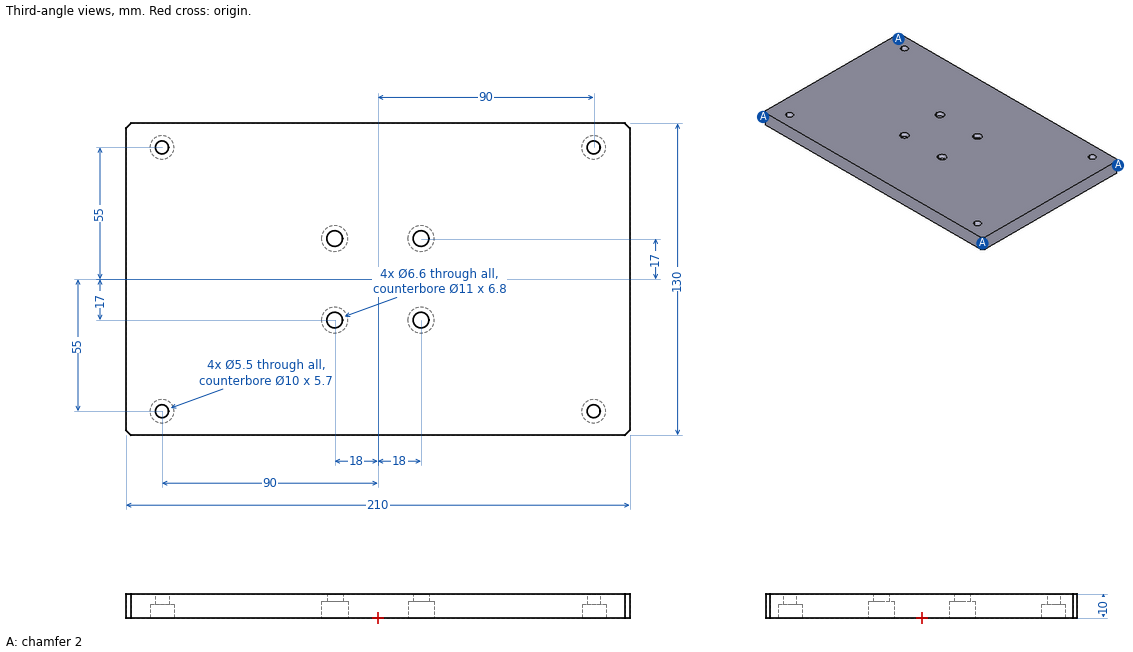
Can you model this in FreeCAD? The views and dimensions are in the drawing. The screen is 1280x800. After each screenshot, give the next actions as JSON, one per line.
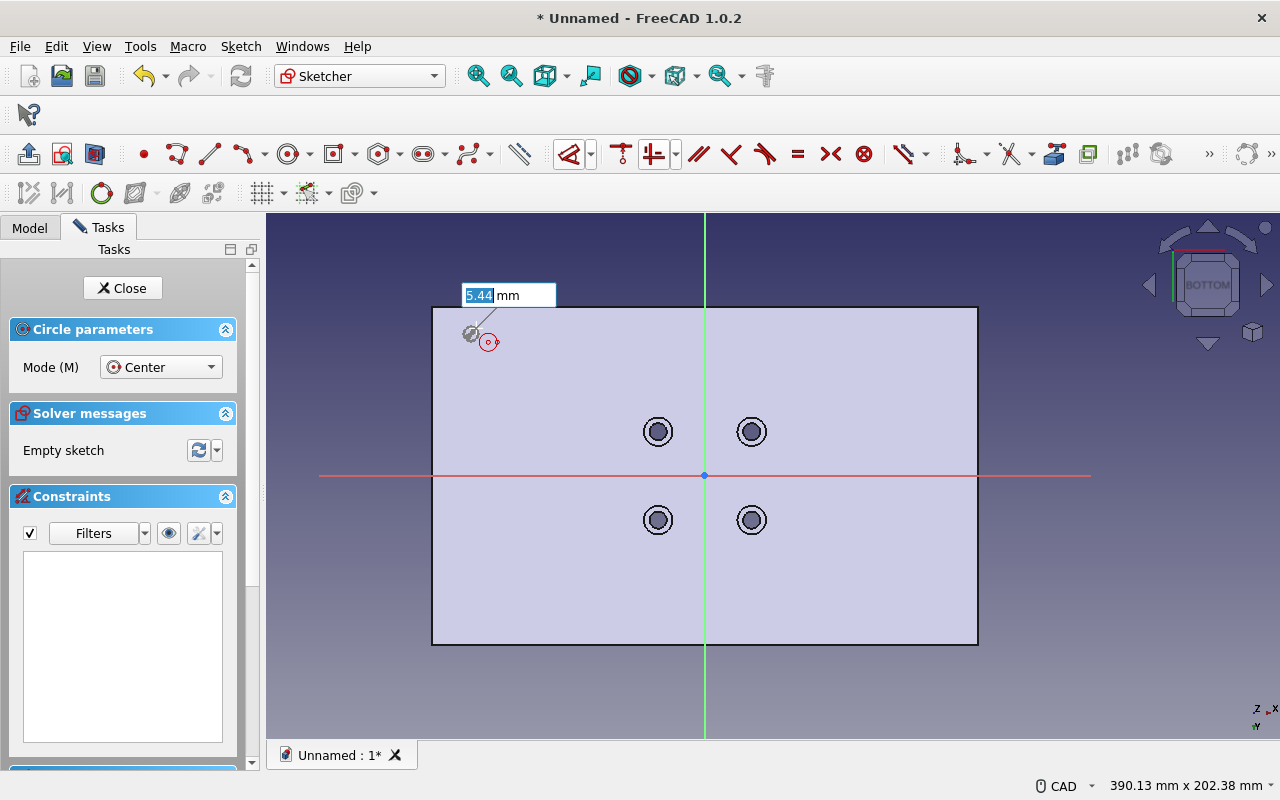
{"action": "type", "text": "5.5"}
{"action": "key", "text": "Return"}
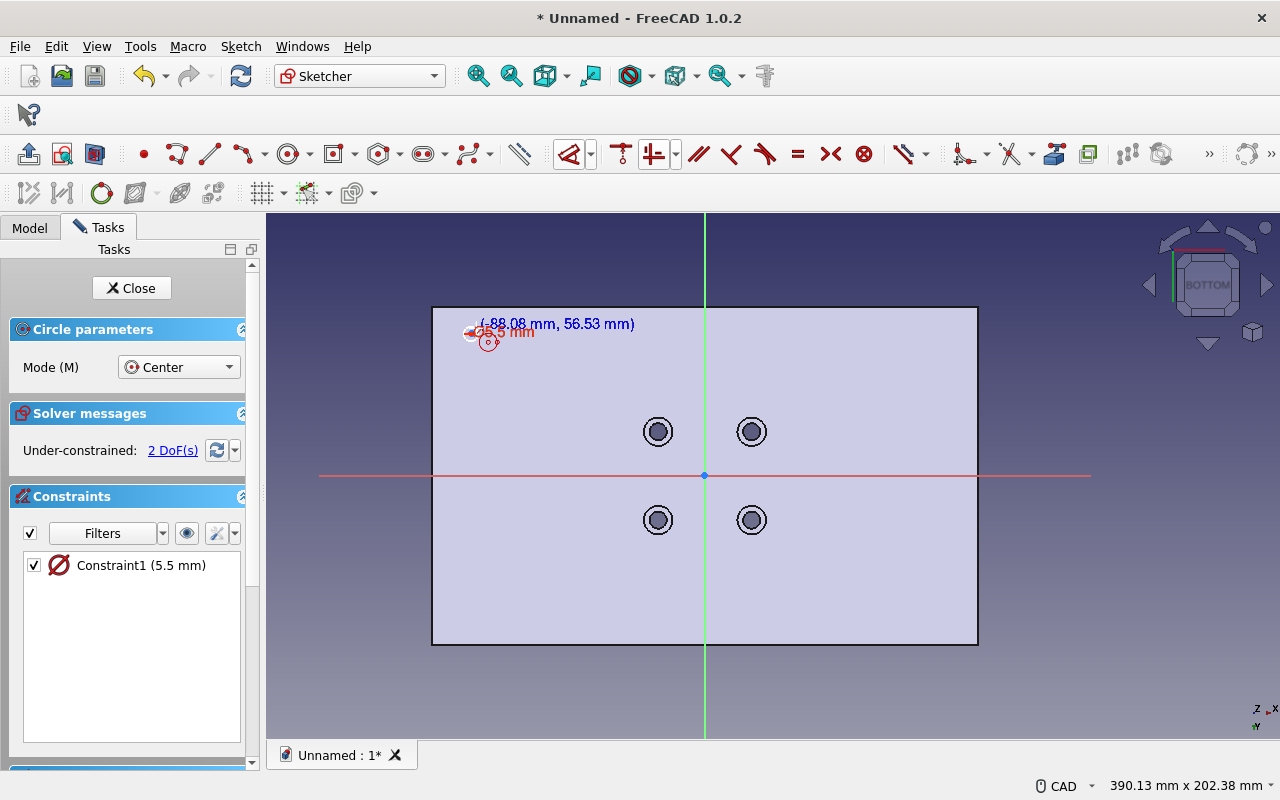
{"action": "scroll", "coordinate": [471, 619], "scroll_direction": "up", "scroll_amount": 6}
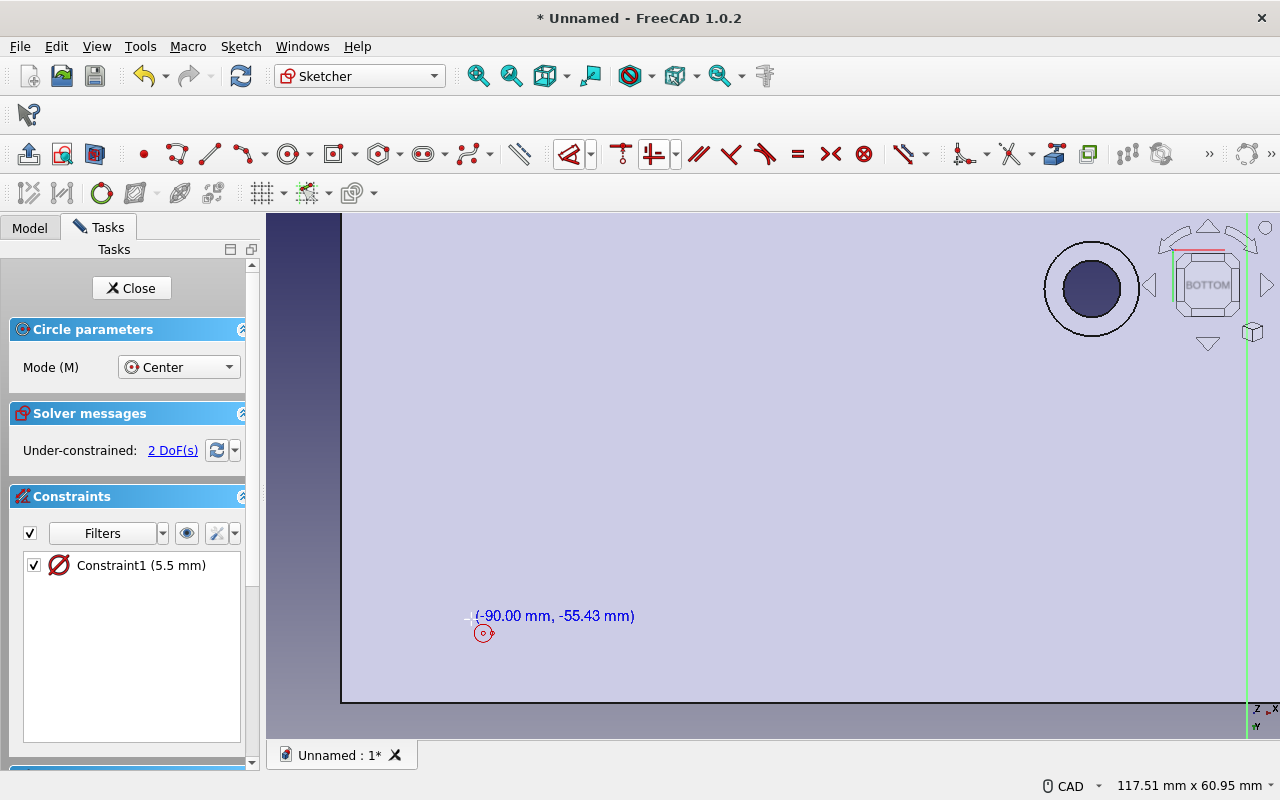
{"action": "scroll", "coordinate": [471, 620], "scroll_direction": "down", "scroll_amount": 6}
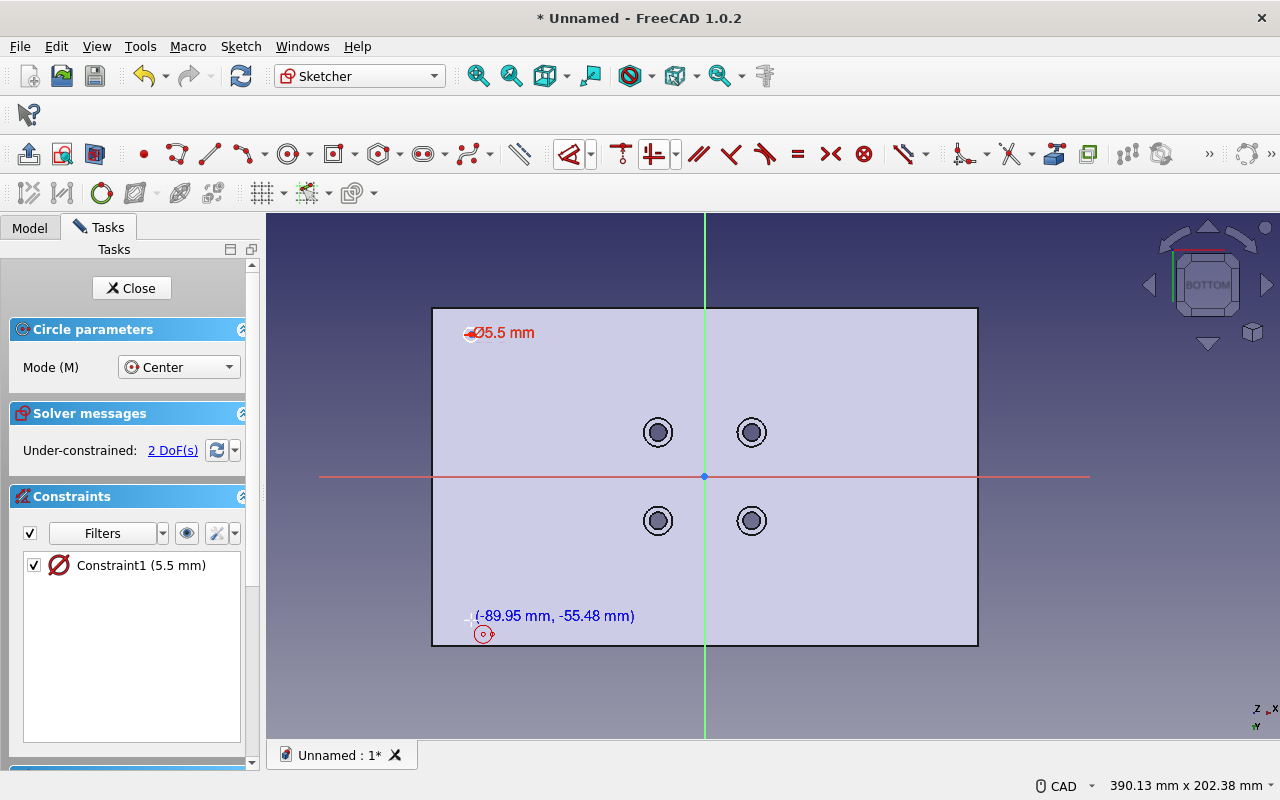
{"action": "left_click", "coordinate": [471, 620]}
{"action": "mouse_move", "coordinate": [476, 615]}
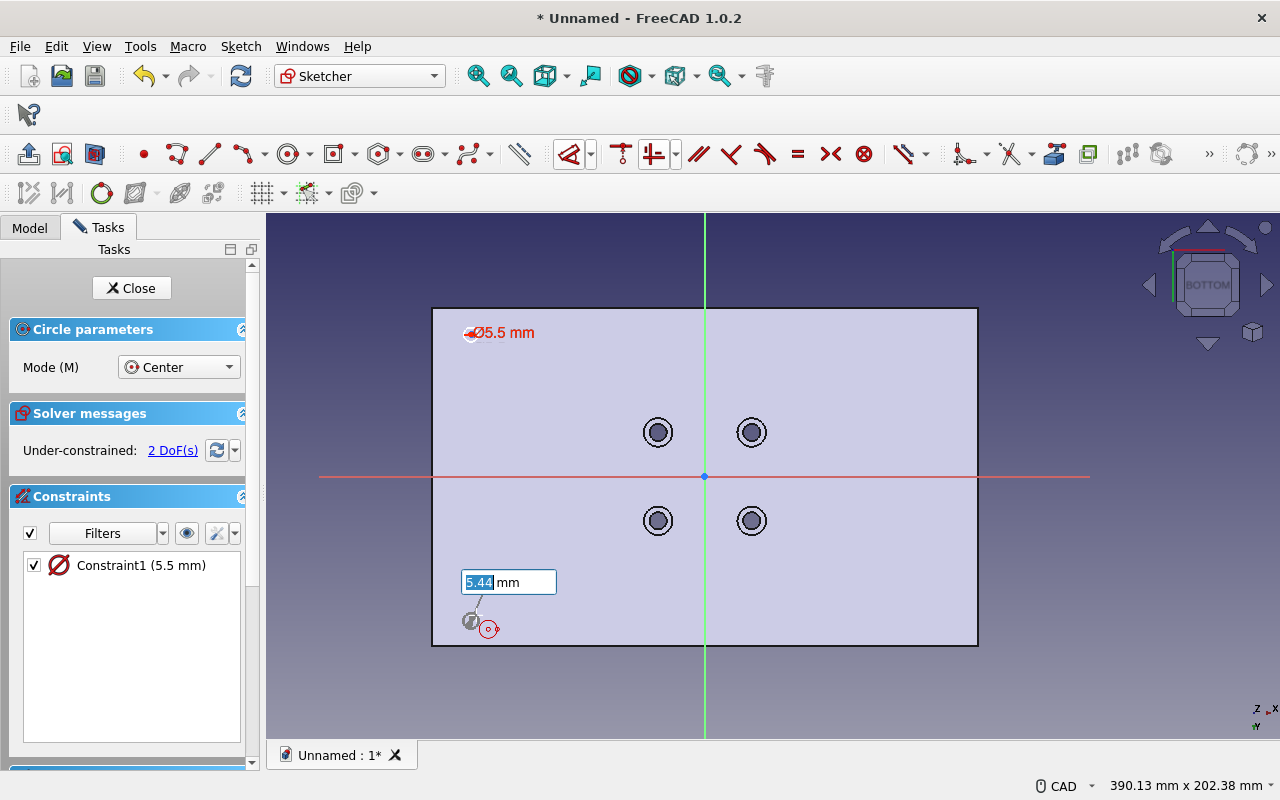
{"action": "type", "text": "5.5"}
{"action": "key", "text": "Return"}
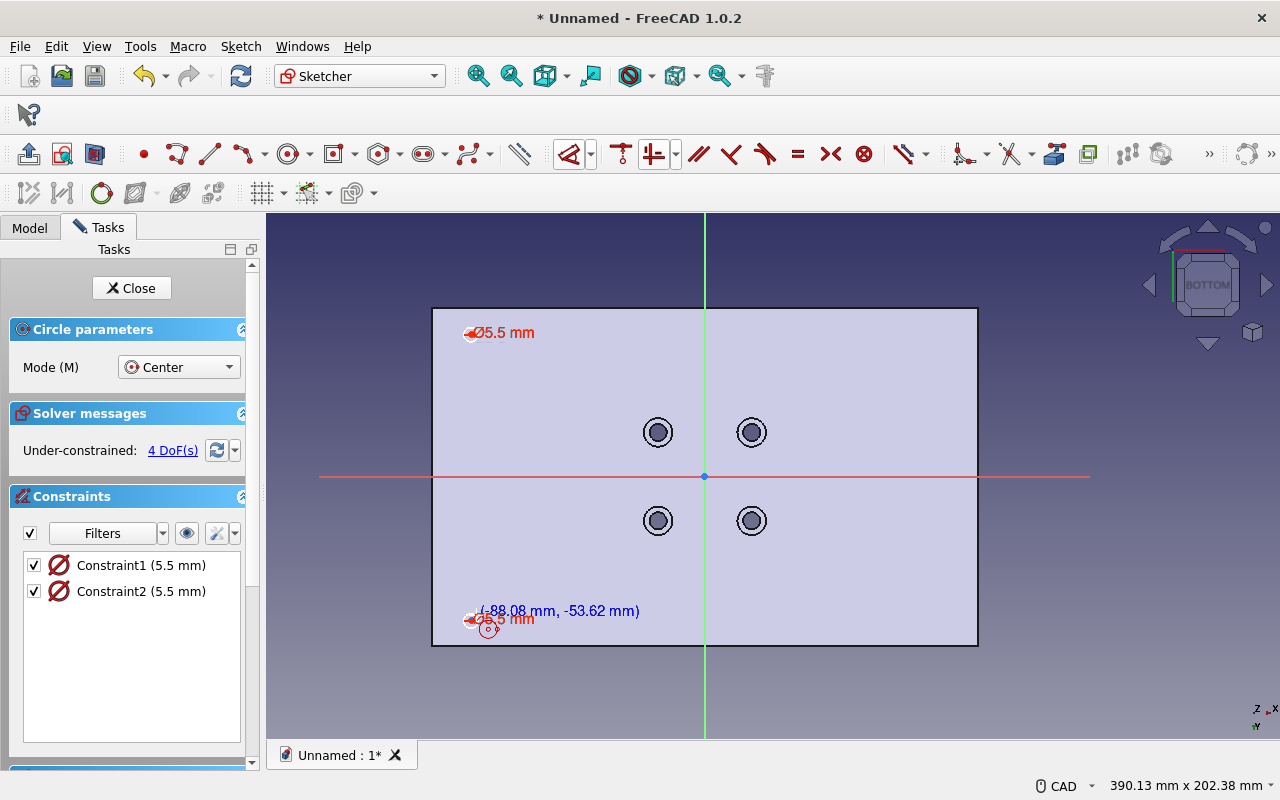
{"action": "scroll", "coordinate": [939, 620], "scroll_direction": "up", "scroll_amount": 6}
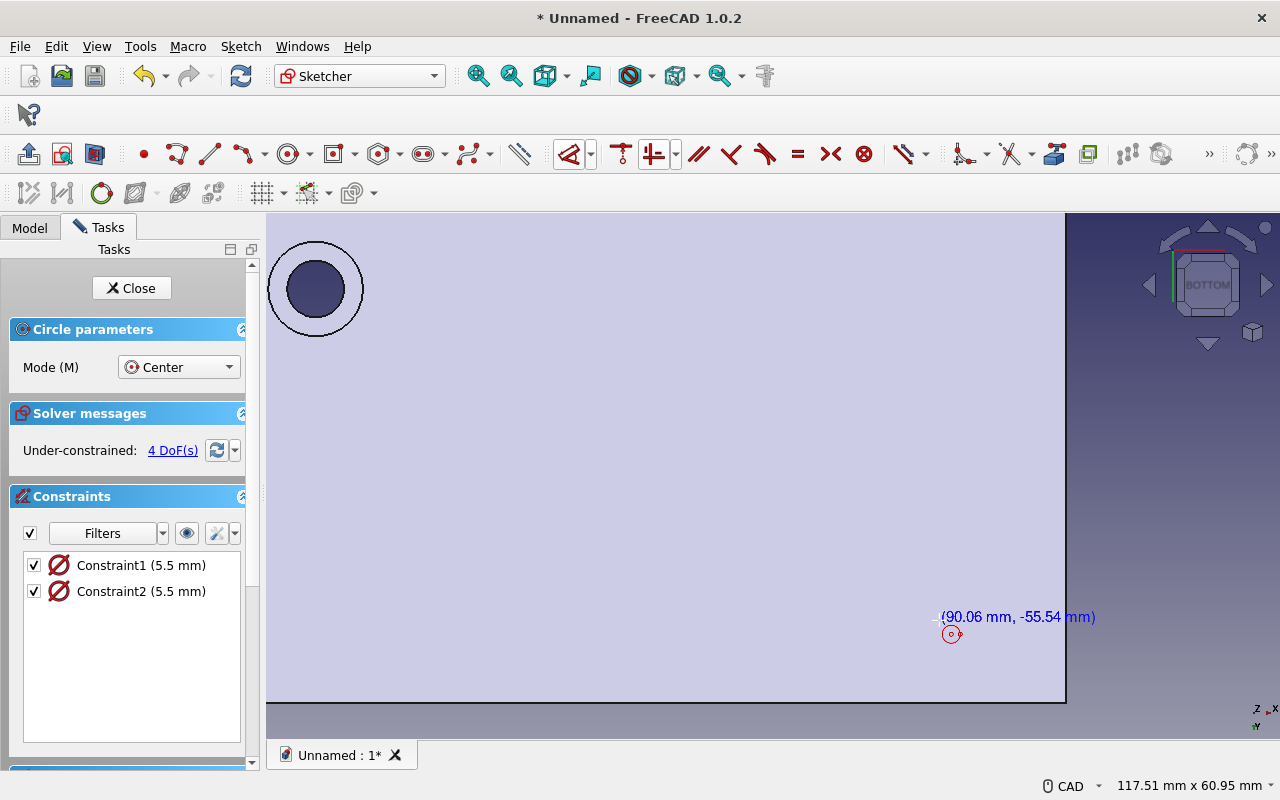
{"action": "scroll", "coordinate": [939, 620], "scroll_direction": "down", "scroll_amount": 6}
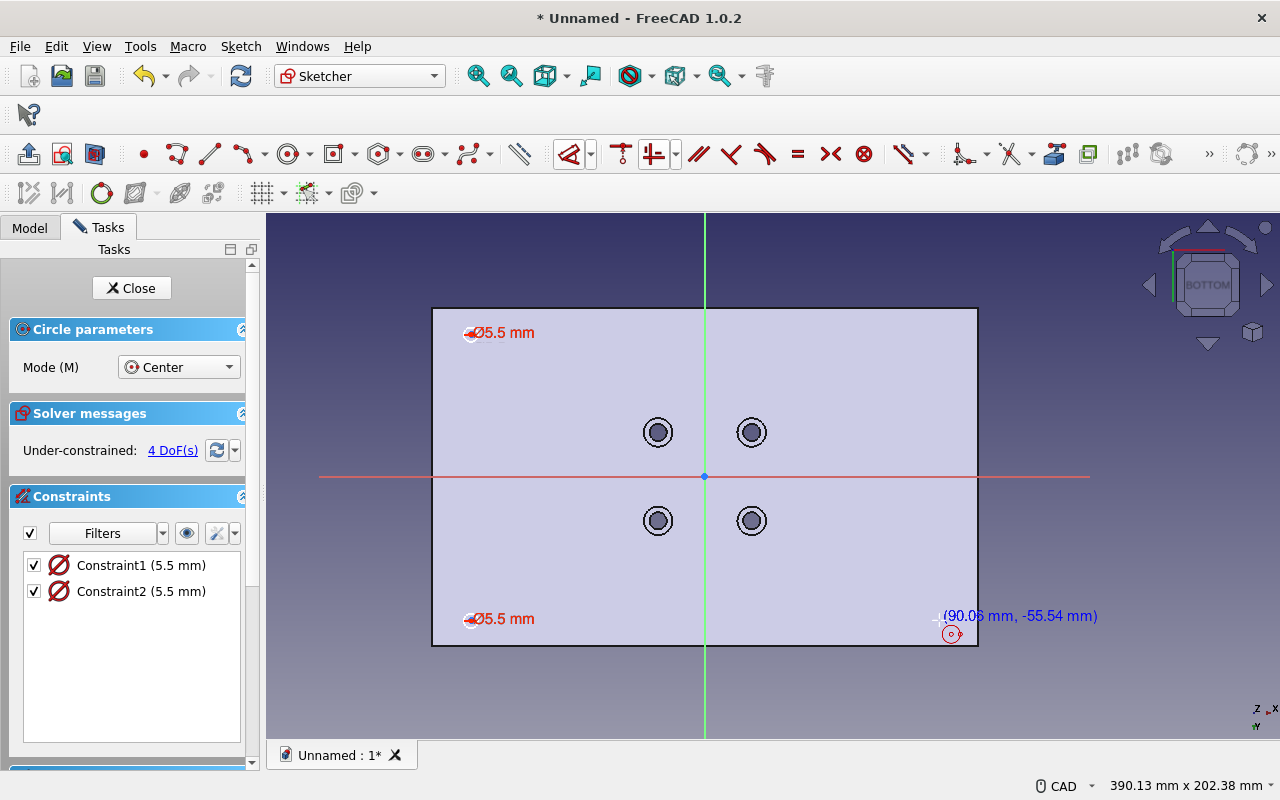
{"action": "left_click", "coordinate": [939, 620]}
{"action": "mouse_move", "coordinate": [944, 615]}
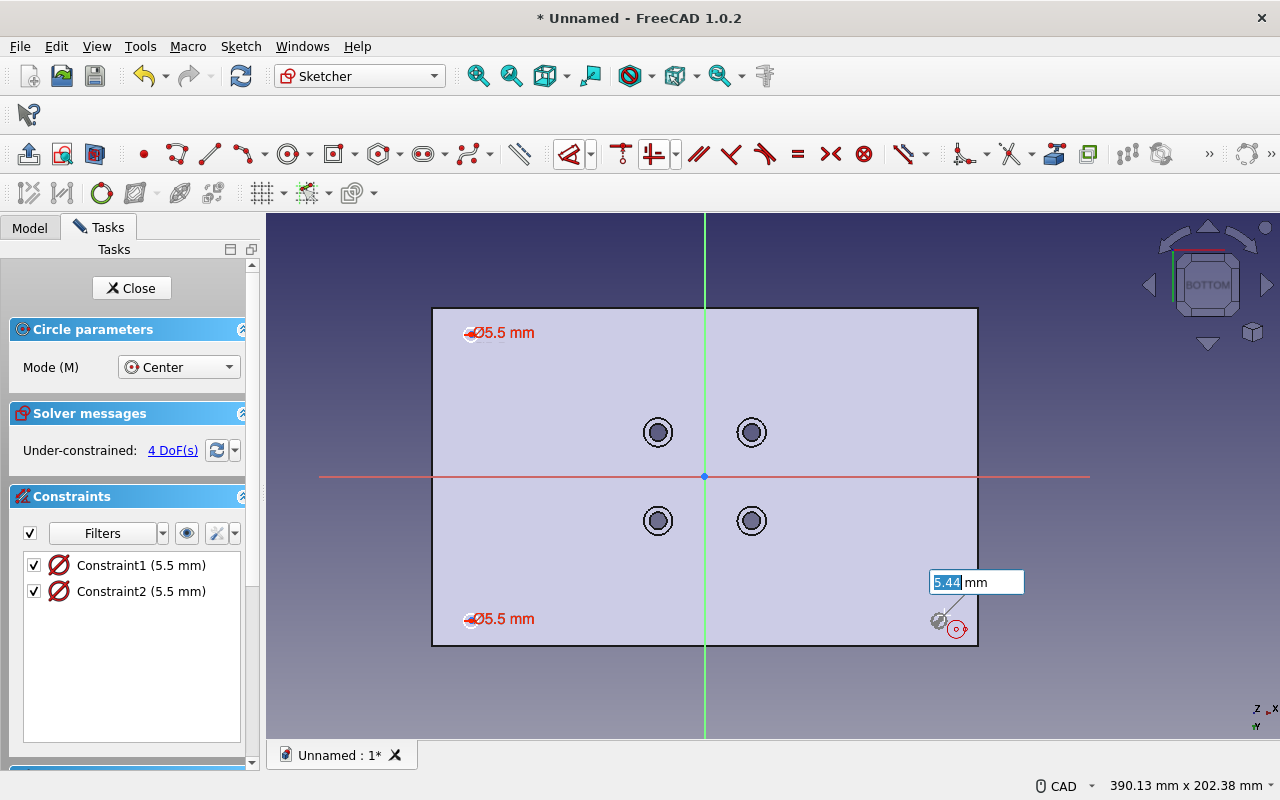
{"action": "type", "text": "5.5"}
{"action": "key", "text": "Return"}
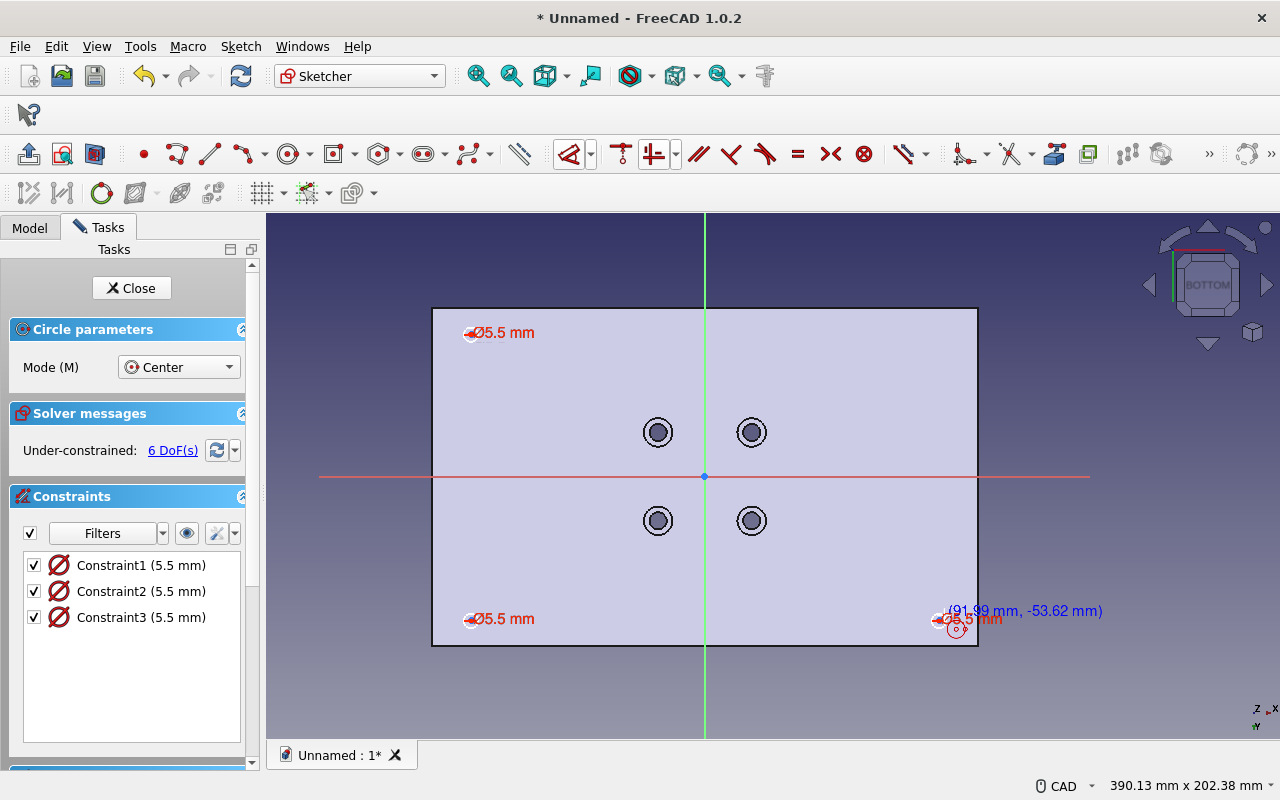
{"action": "scroll", "coordinate": [939, 334], "scroll_direction": "up", "scroll_amount": 6}